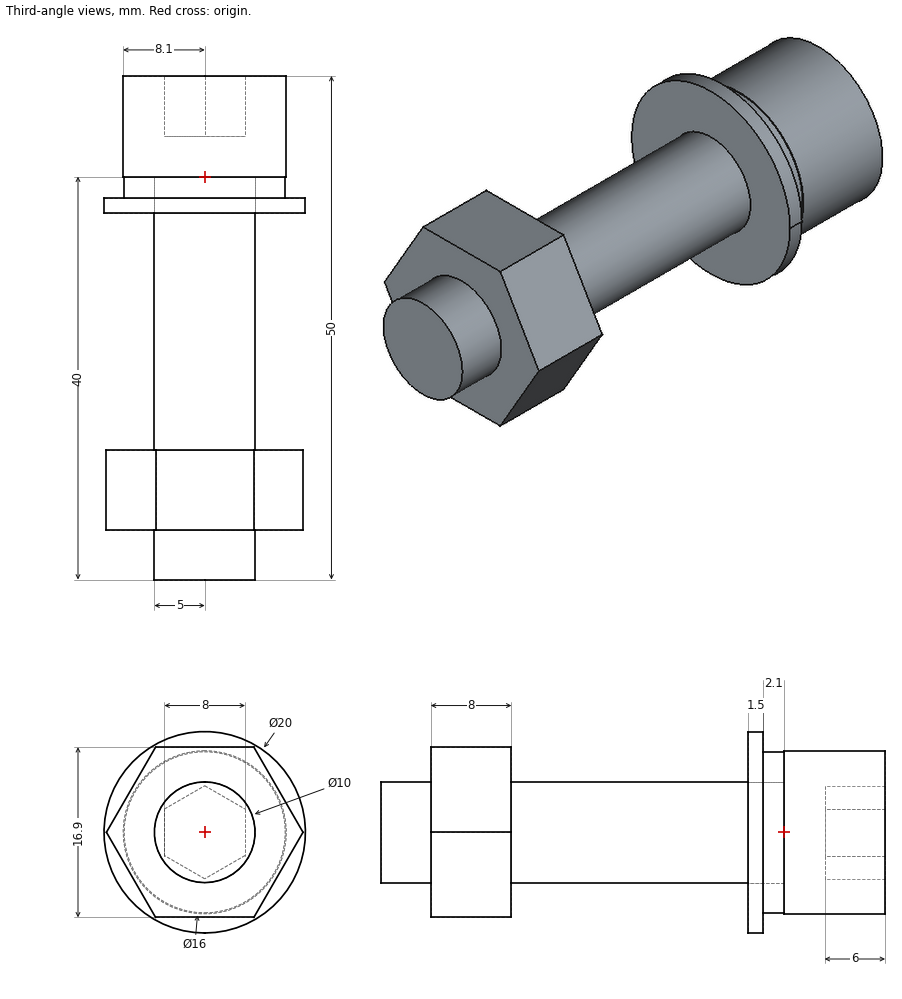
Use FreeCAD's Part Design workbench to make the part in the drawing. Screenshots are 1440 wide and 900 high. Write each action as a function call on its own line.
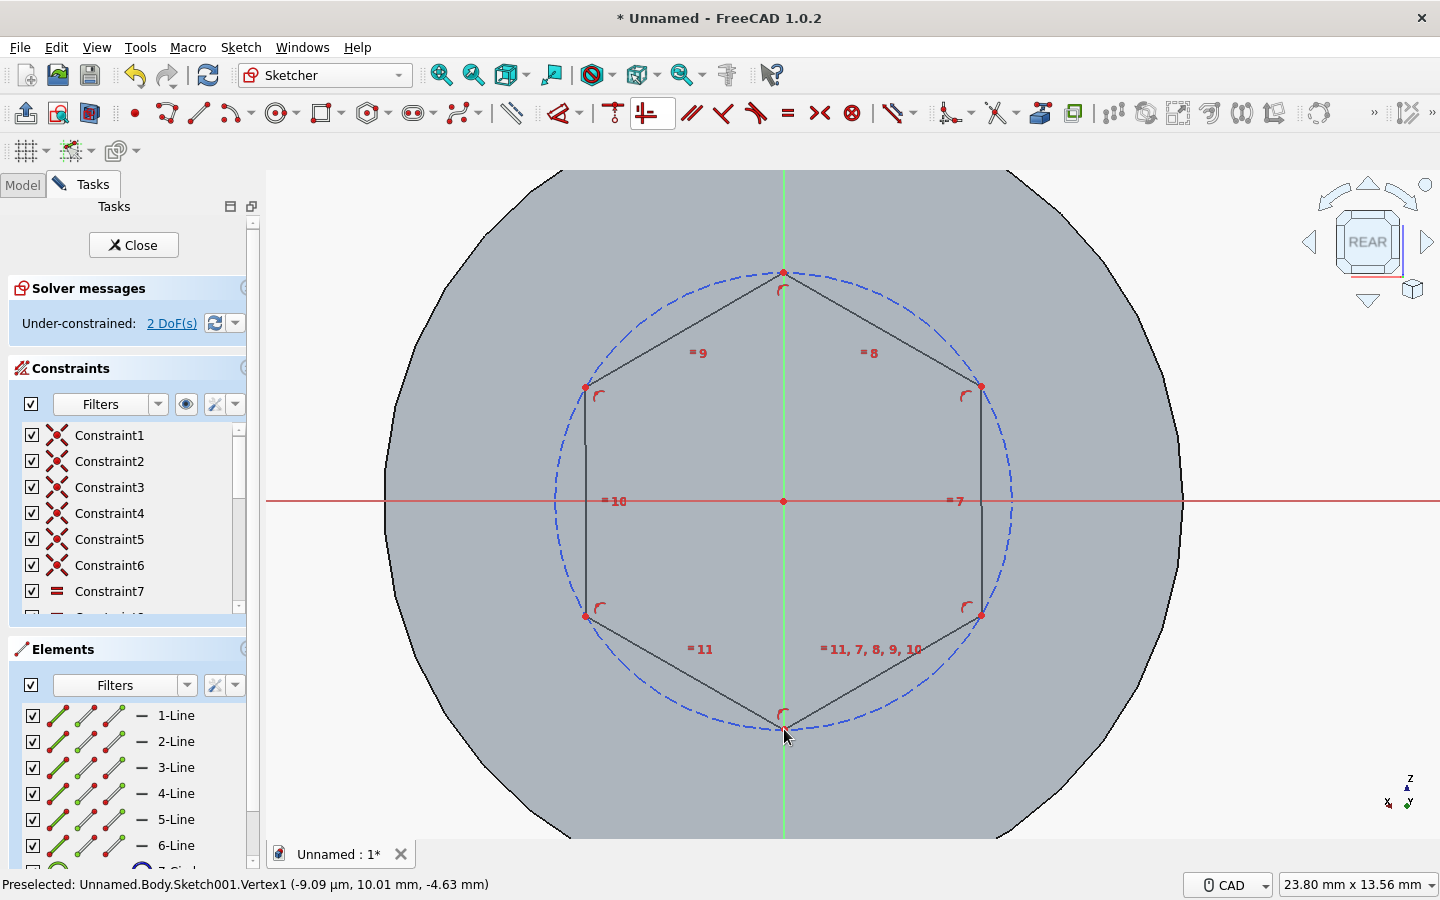
click(982, 547)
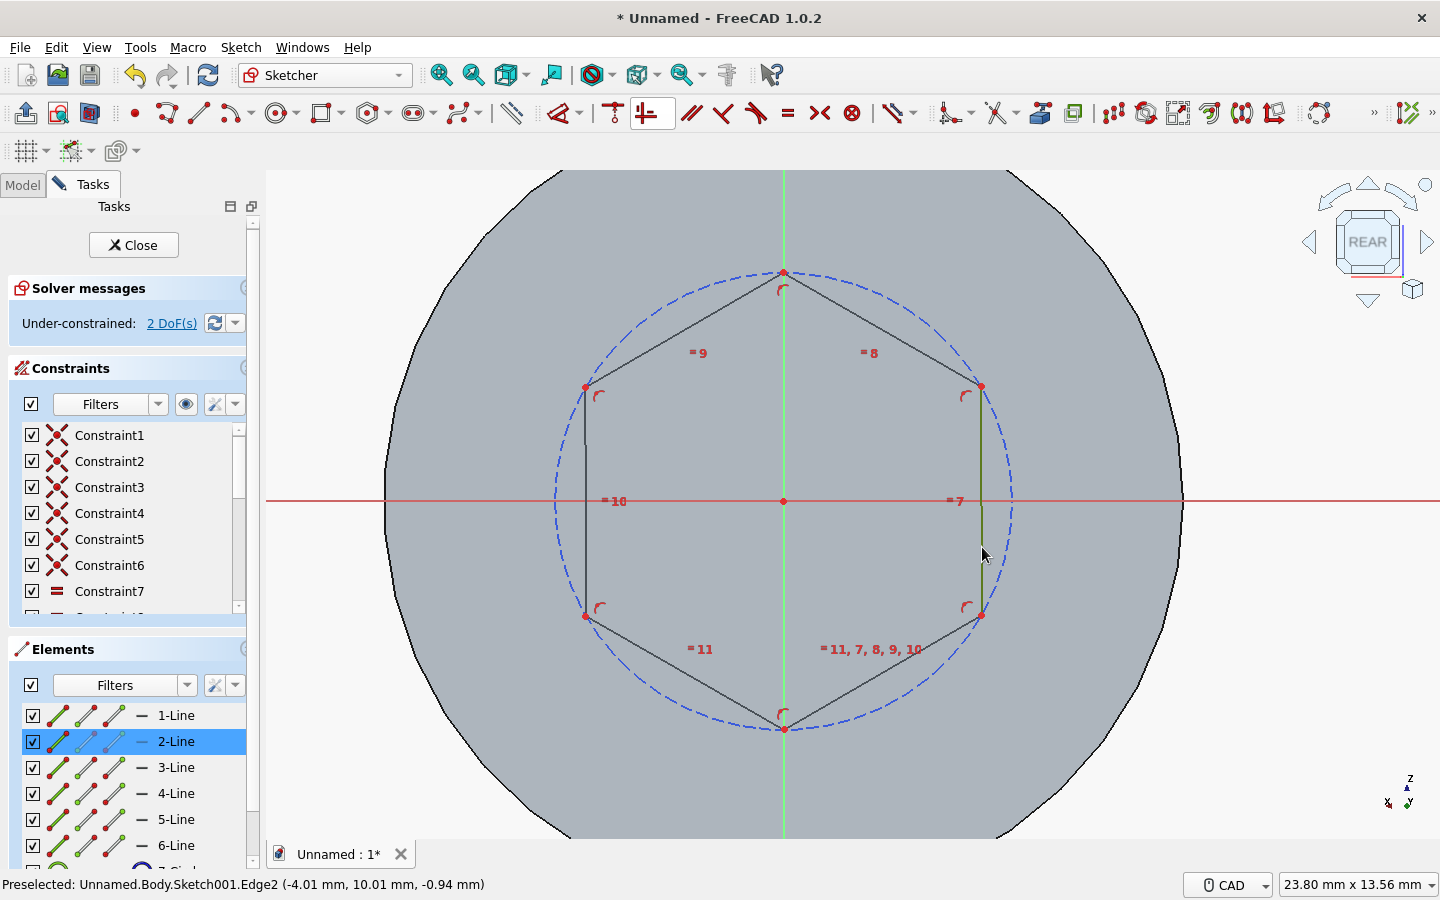
click(670, 114)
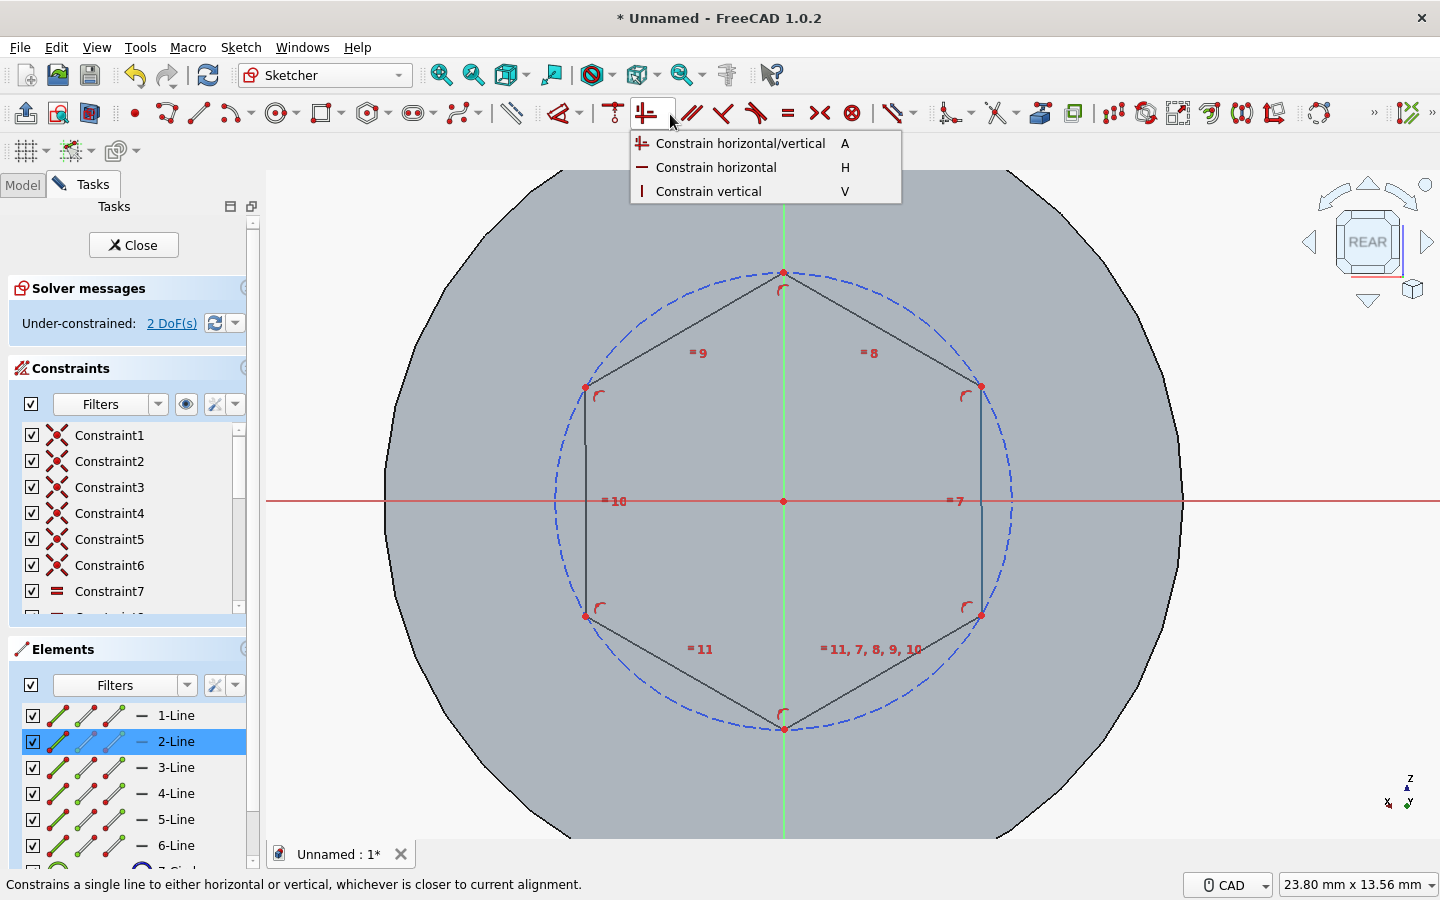
click(766, 191)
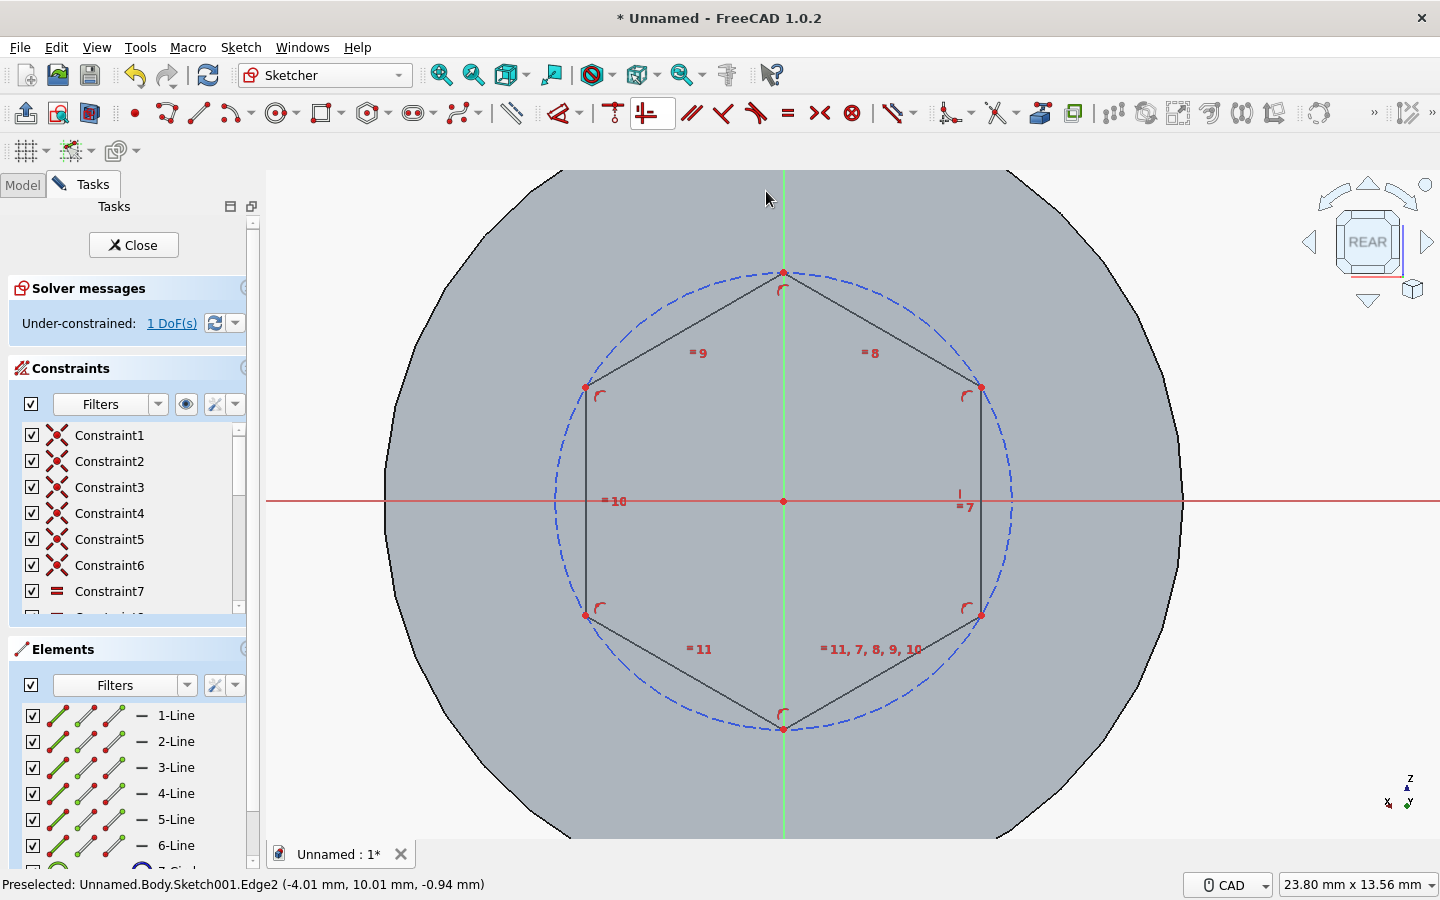
click(558, 114)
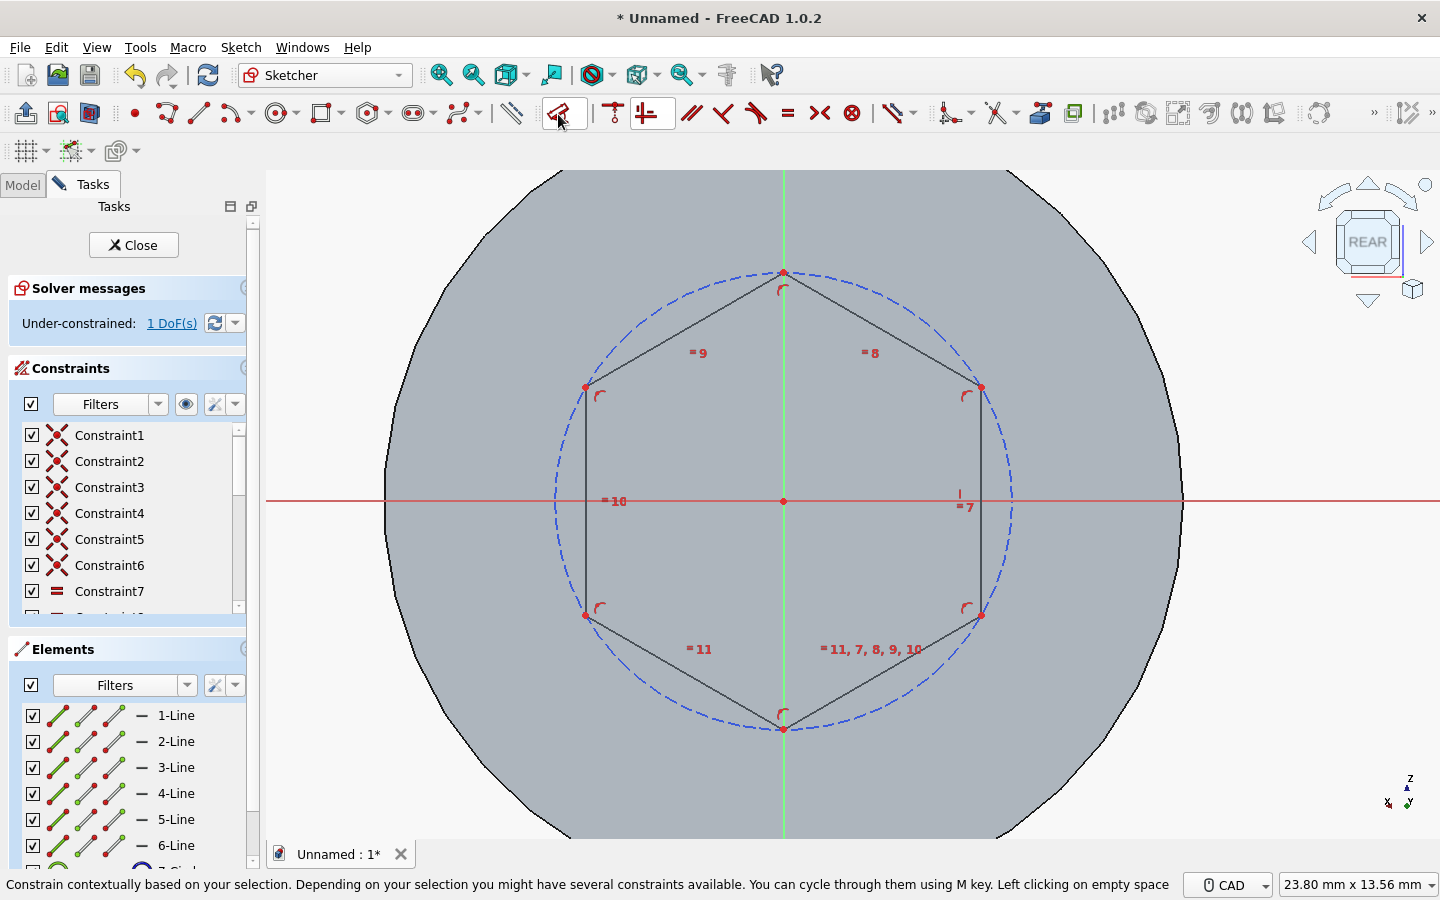
click(586, 387)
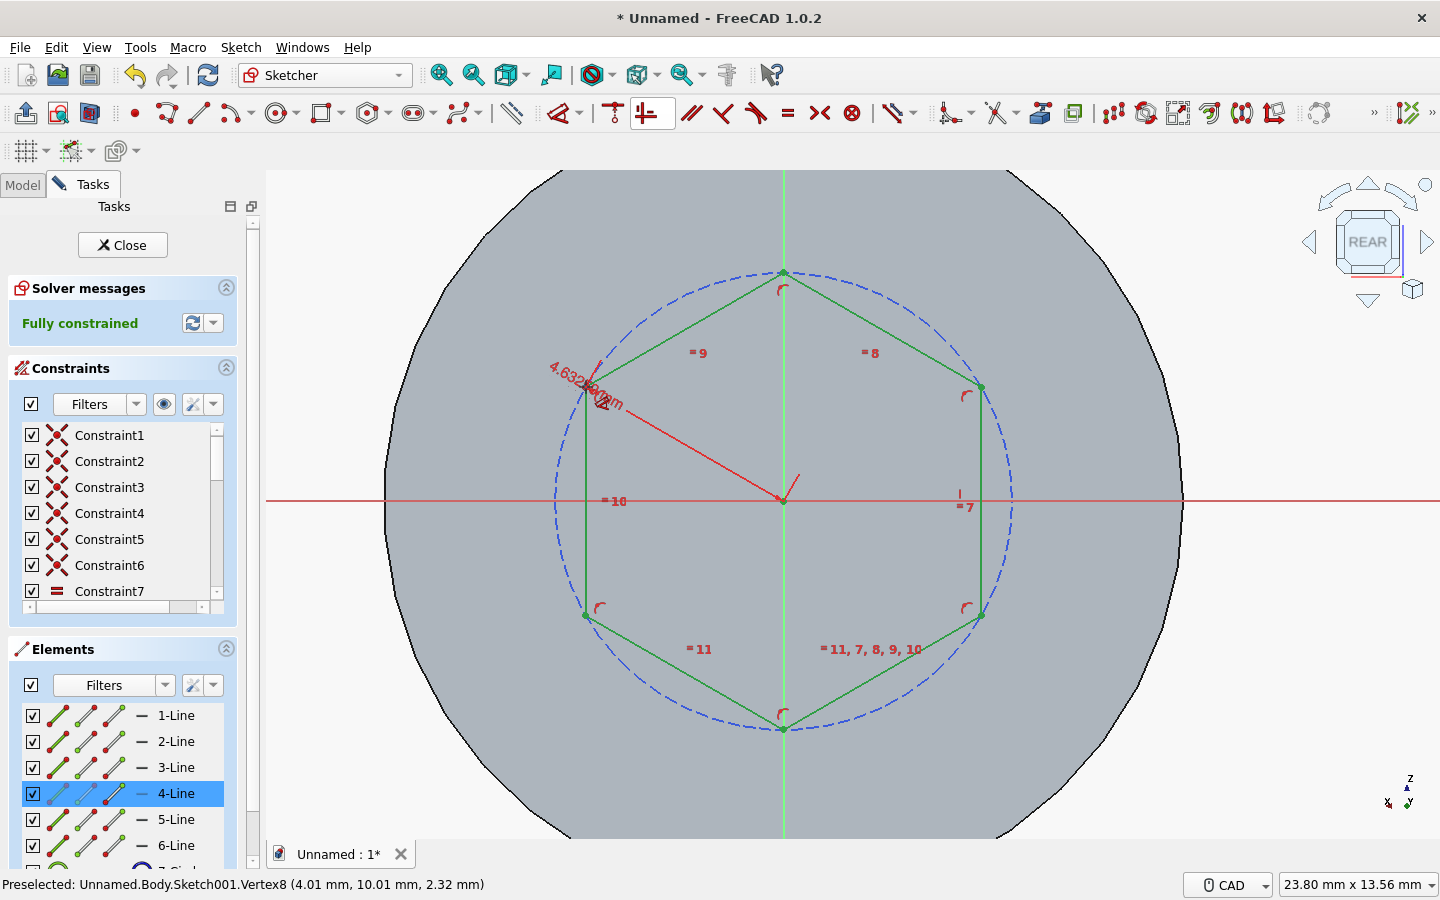
click(981, 616)
click(692, 650)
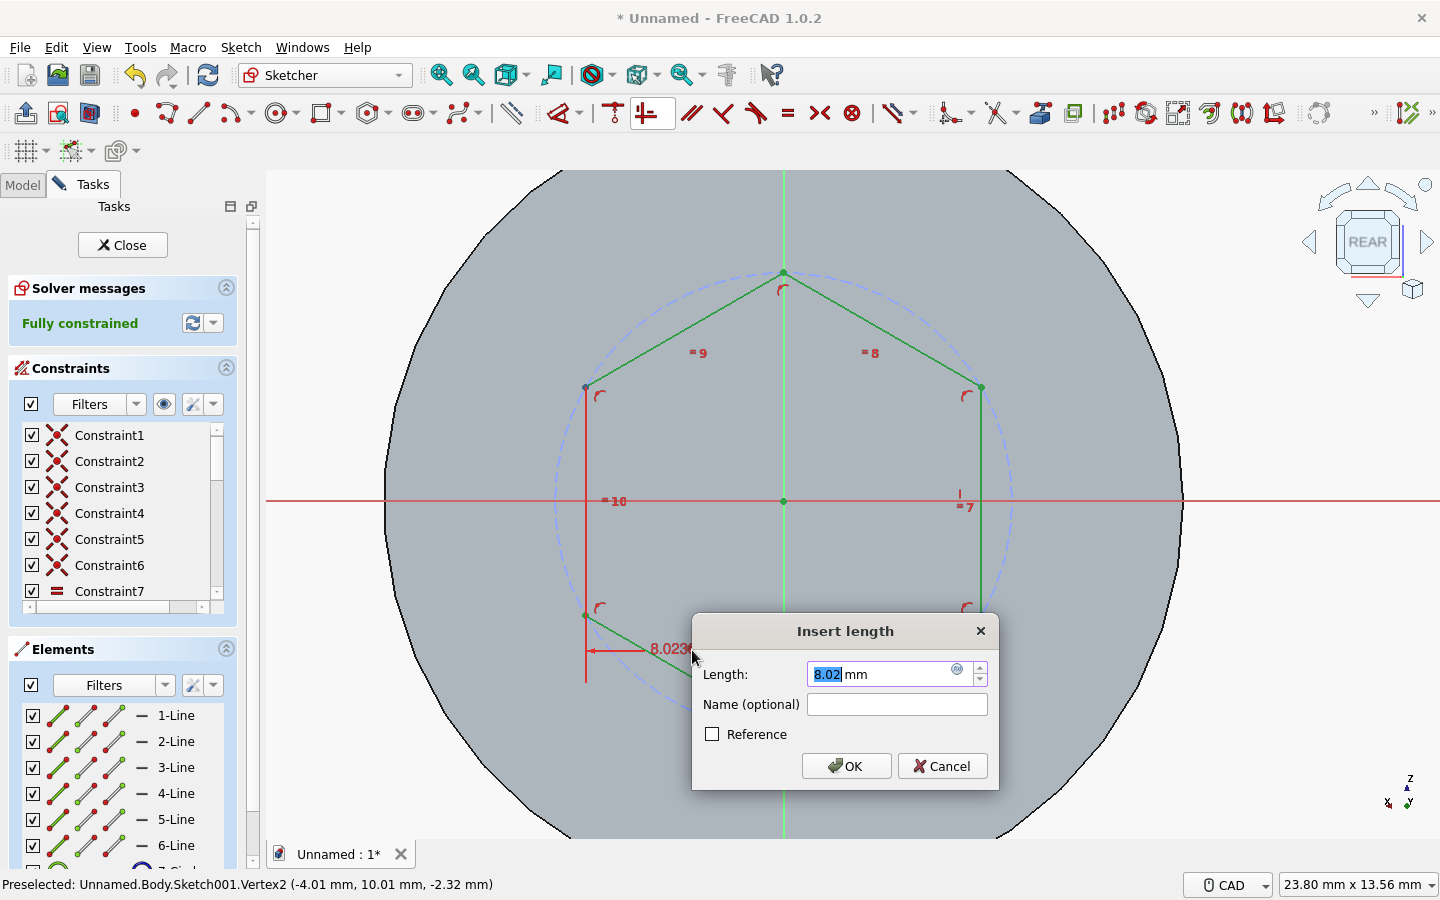
text(8)
key(Return)
key(Escape)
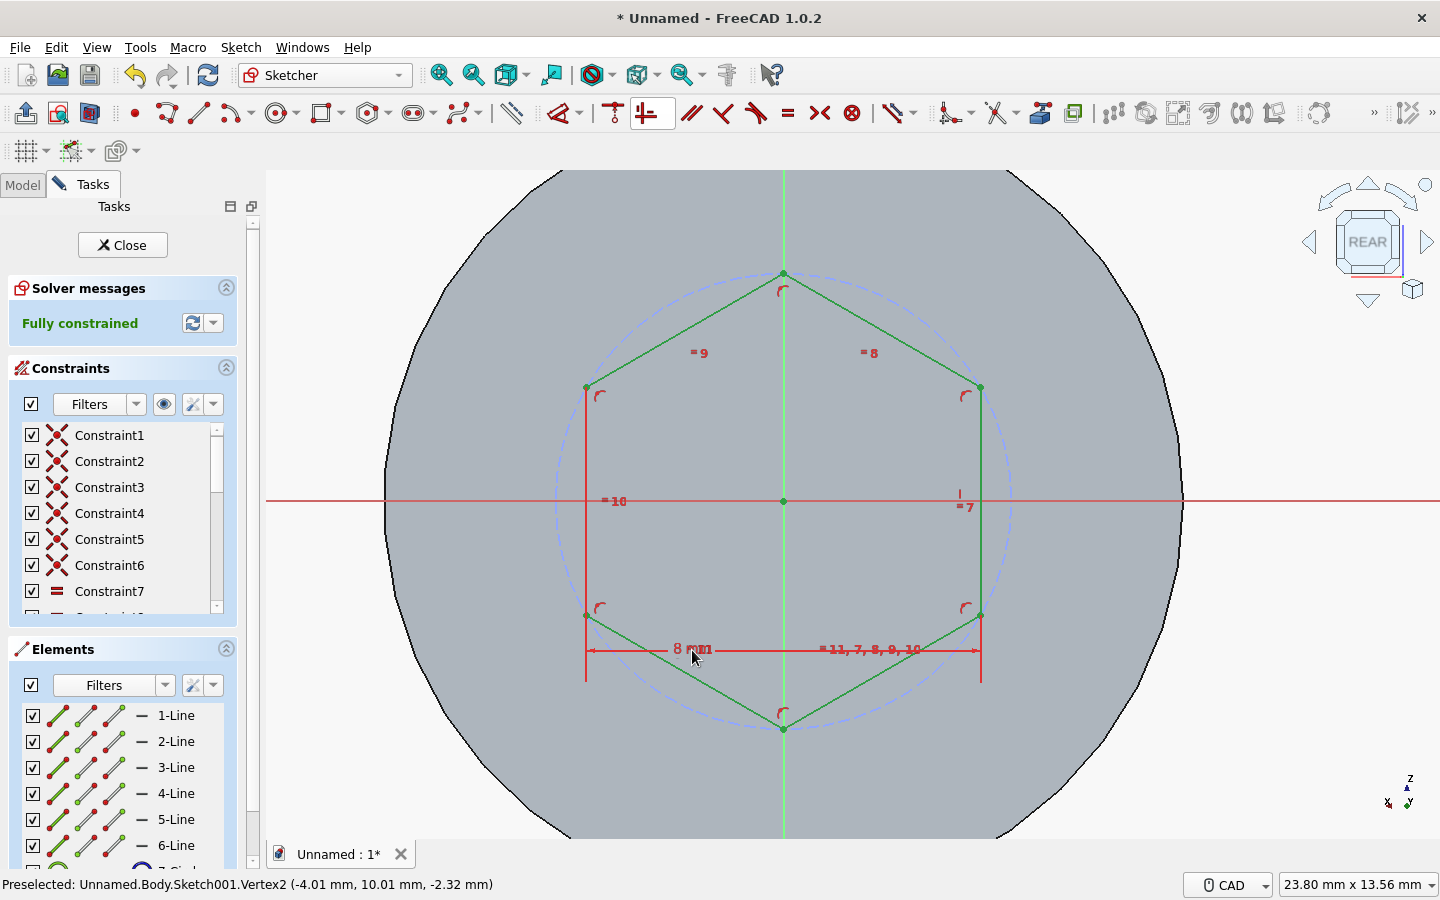
click(123, 245)